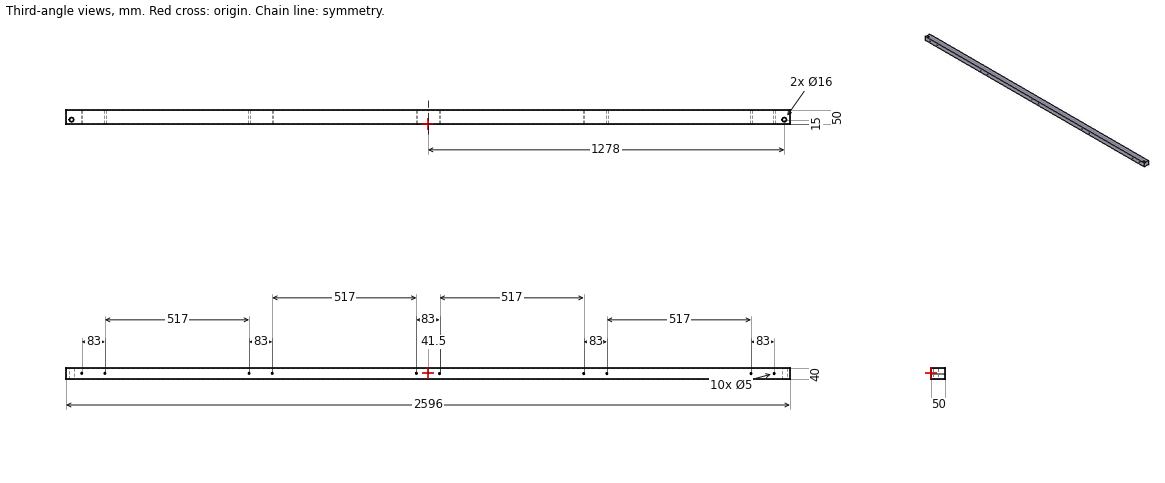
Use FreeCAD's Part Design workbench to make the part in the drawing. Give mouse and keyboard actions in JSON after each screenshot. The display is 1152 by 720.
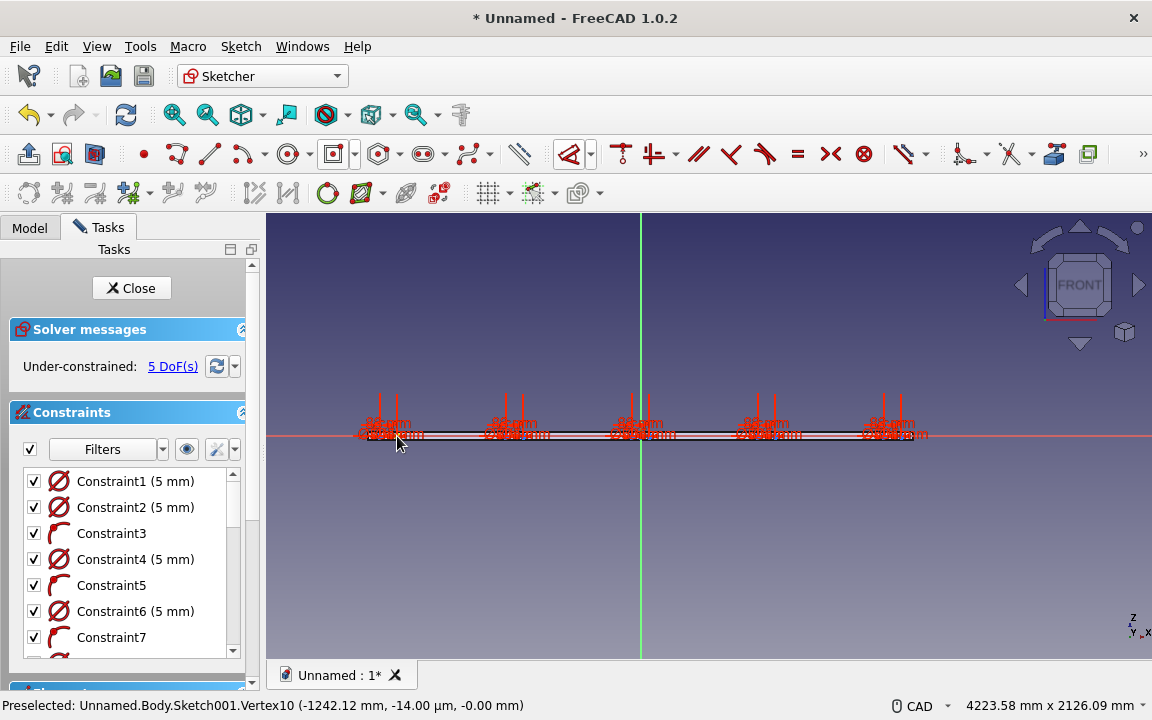
{"action": "scroll", "coordinate": [649, 436], "scroll_direction": "up", "scroll_amount": 8}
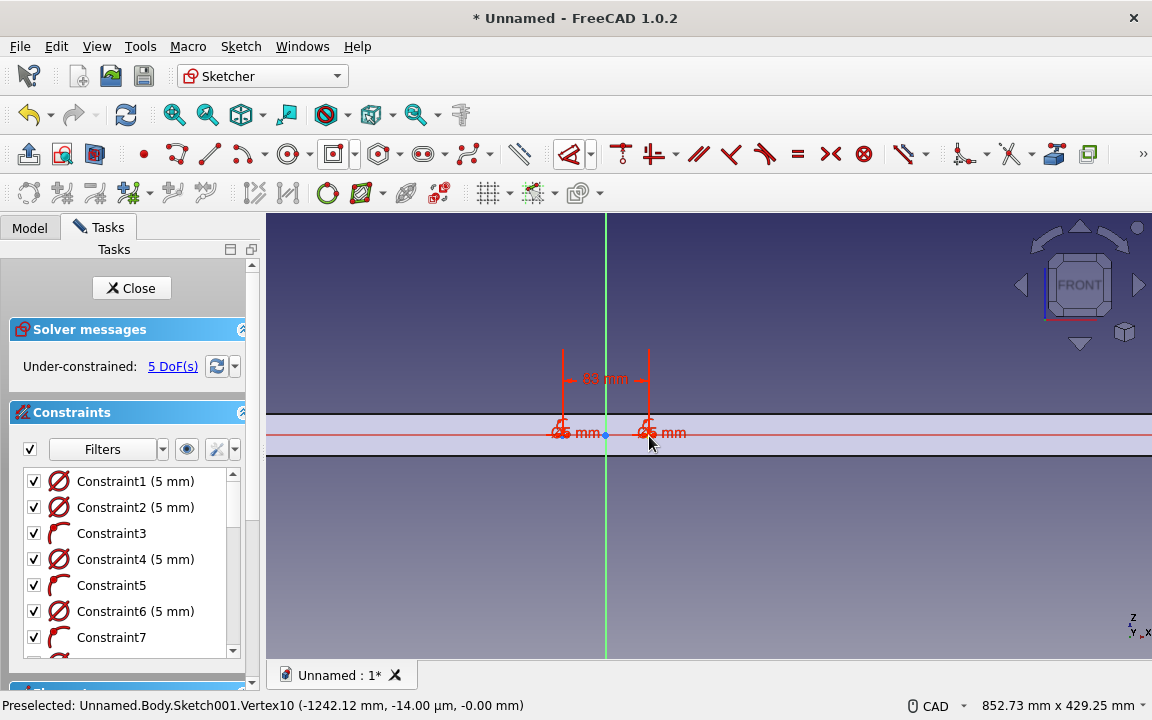
{"action": "left_click", "coordinate": [649, 435]}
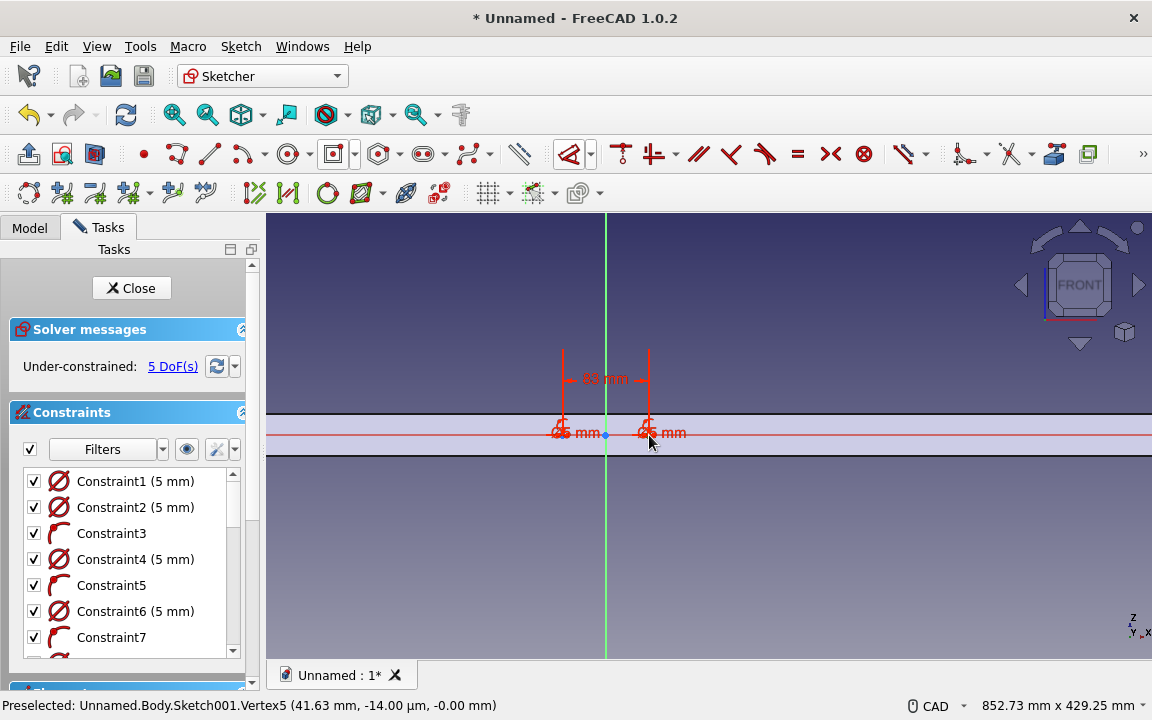
{"action": "left_click", "coordinate": [590, 154]}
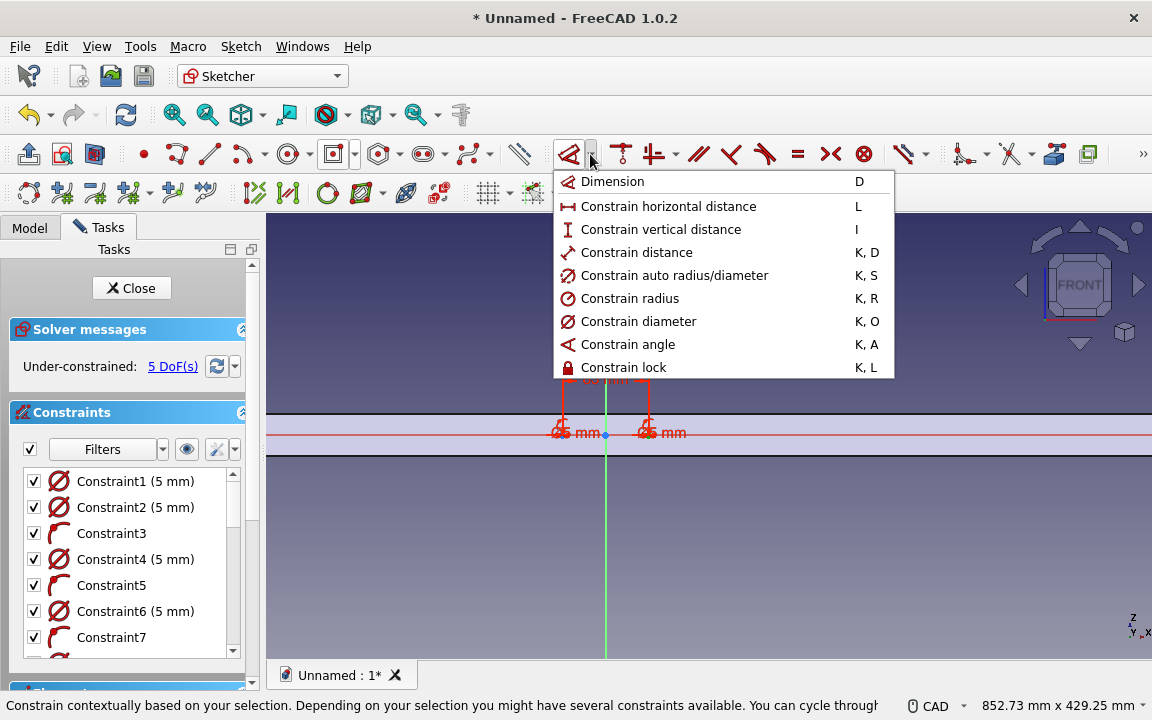
{"action": "left_click", "coordinate": [724, 206]}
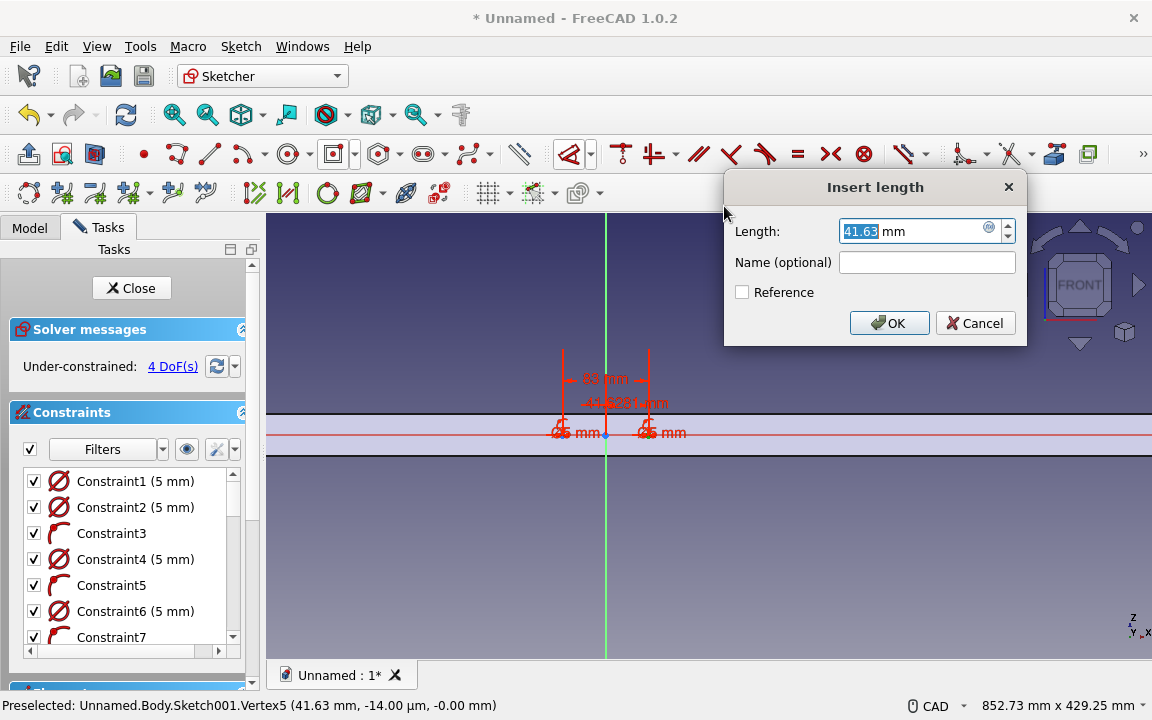
{"action": "type", "text": "41.5"}
{"action": "key", "text": "Return"}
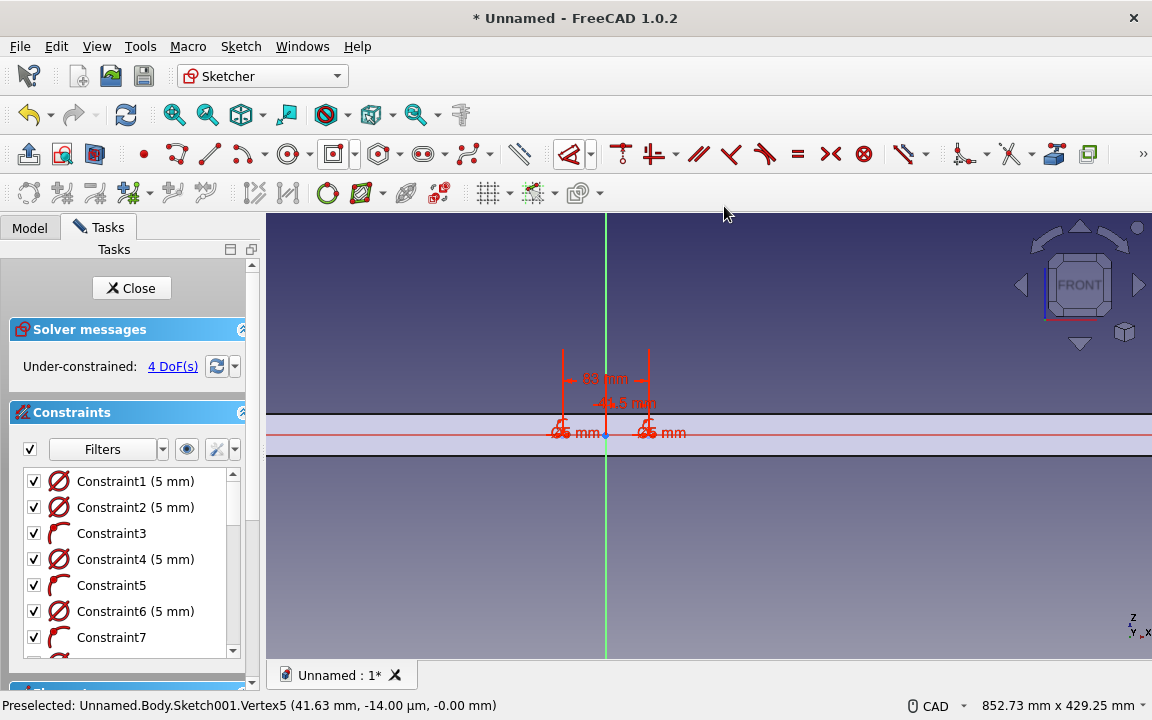
{"action": "scroll", "coordinate": [649, 436], "scroll_direction": "down", "scroll_amount": 8}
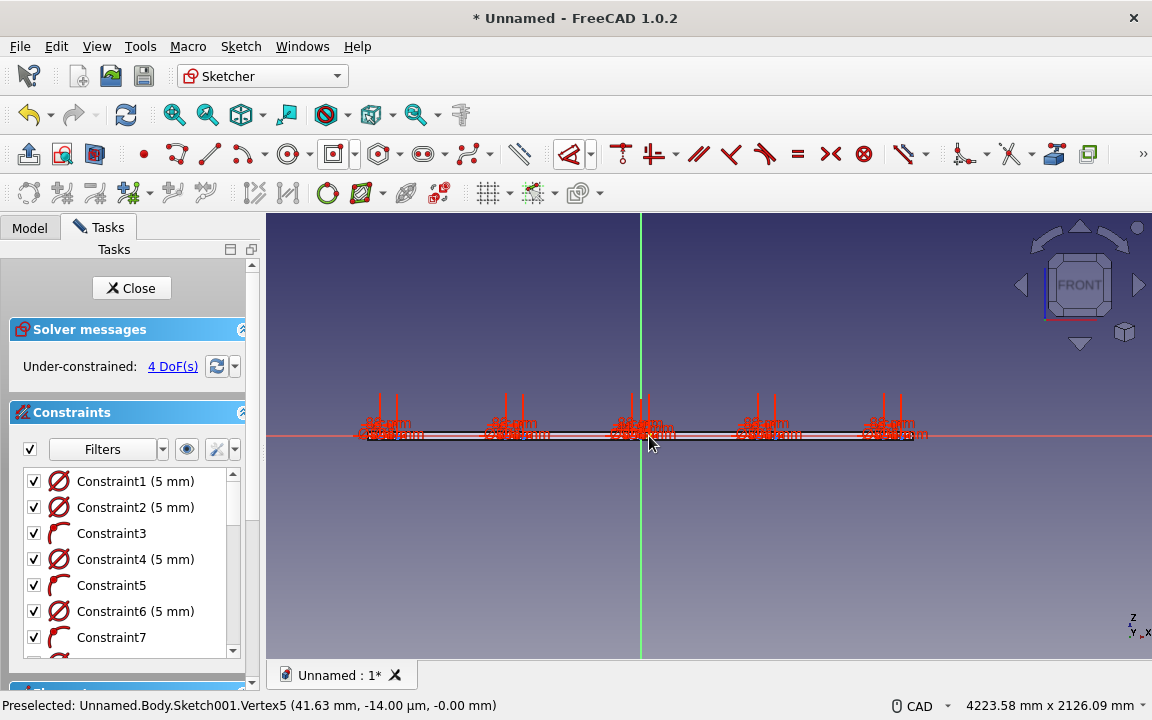
{"action": "left_click", "coordinate": [884, 436]}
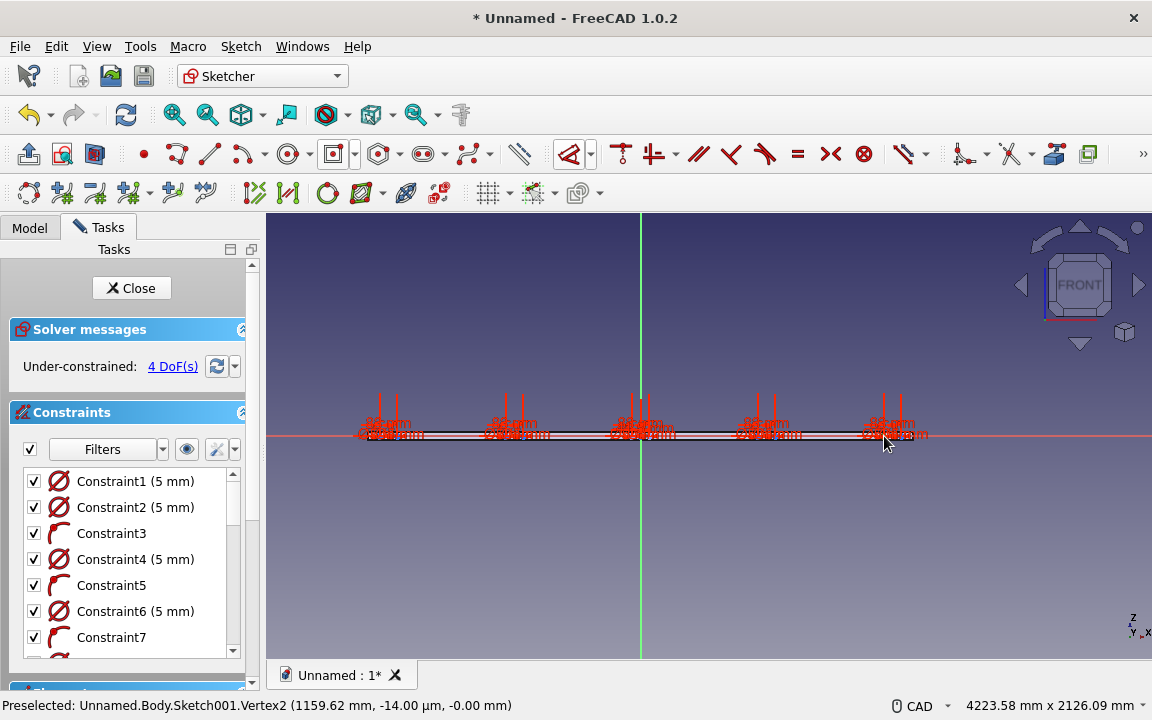
{"action": "left_click", "coordinate": [775, 436]}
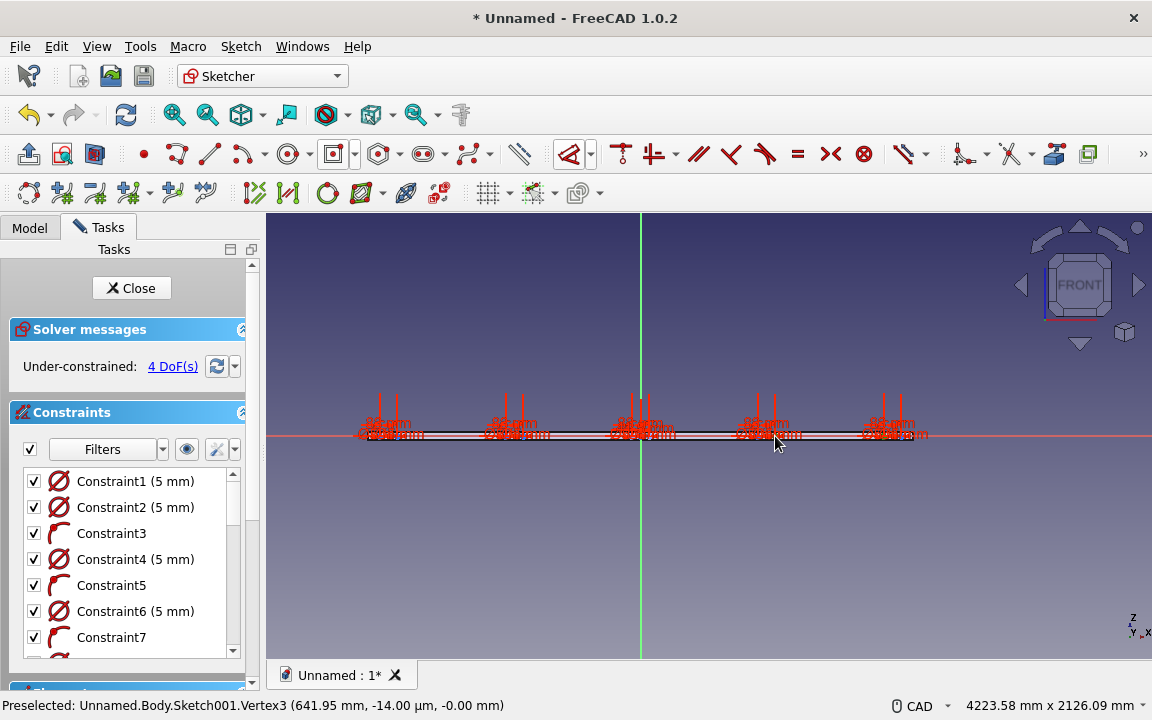
{"action": "left_click", "coordinate": [590, 154]}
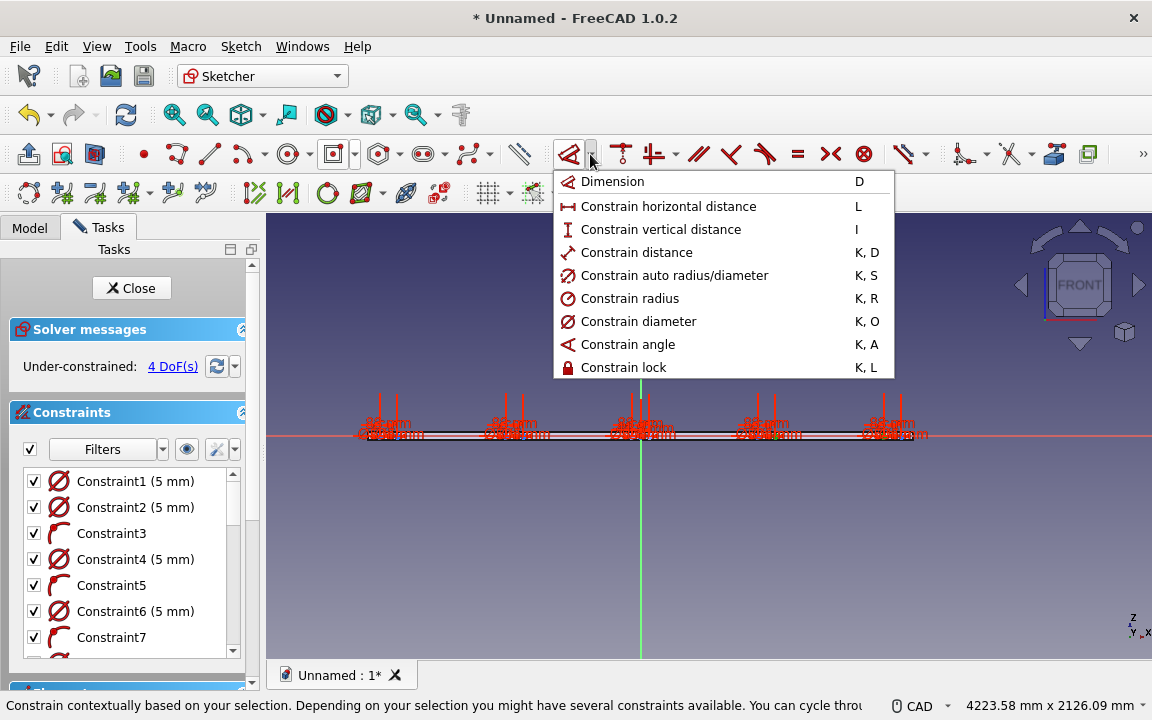
{"action": "left_click", "coordinate": [724, 206]}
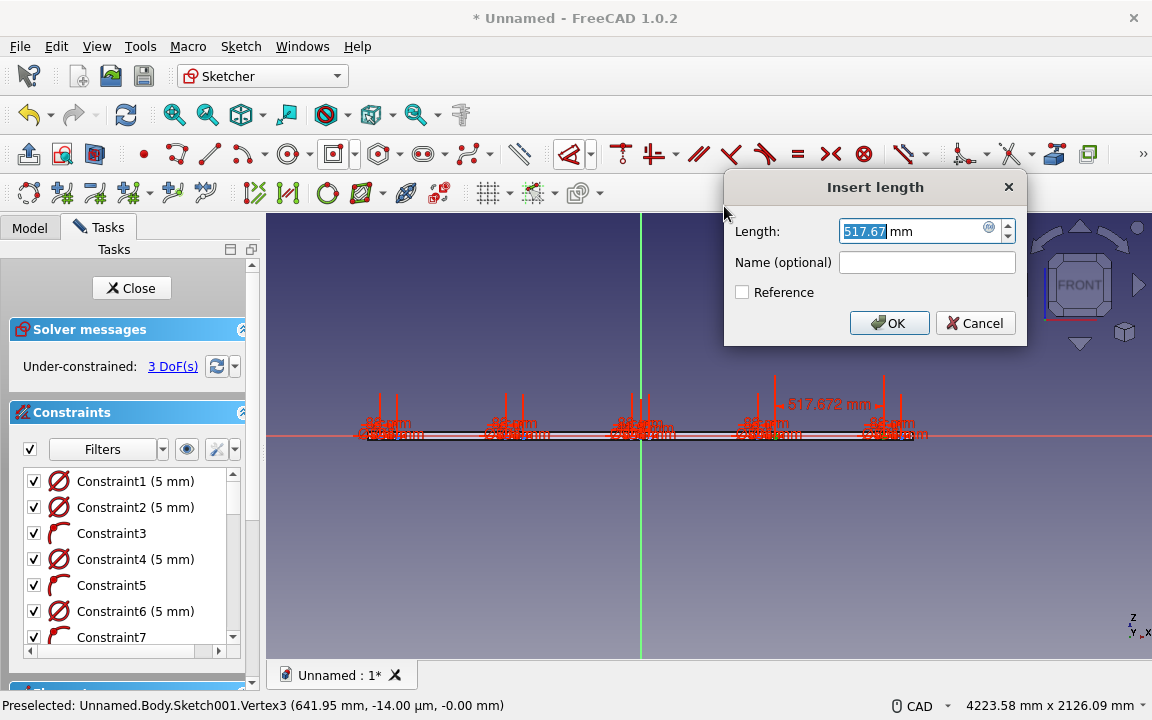
{"action": "type", "text": "517"}
{"action": "key", "text": "Return"}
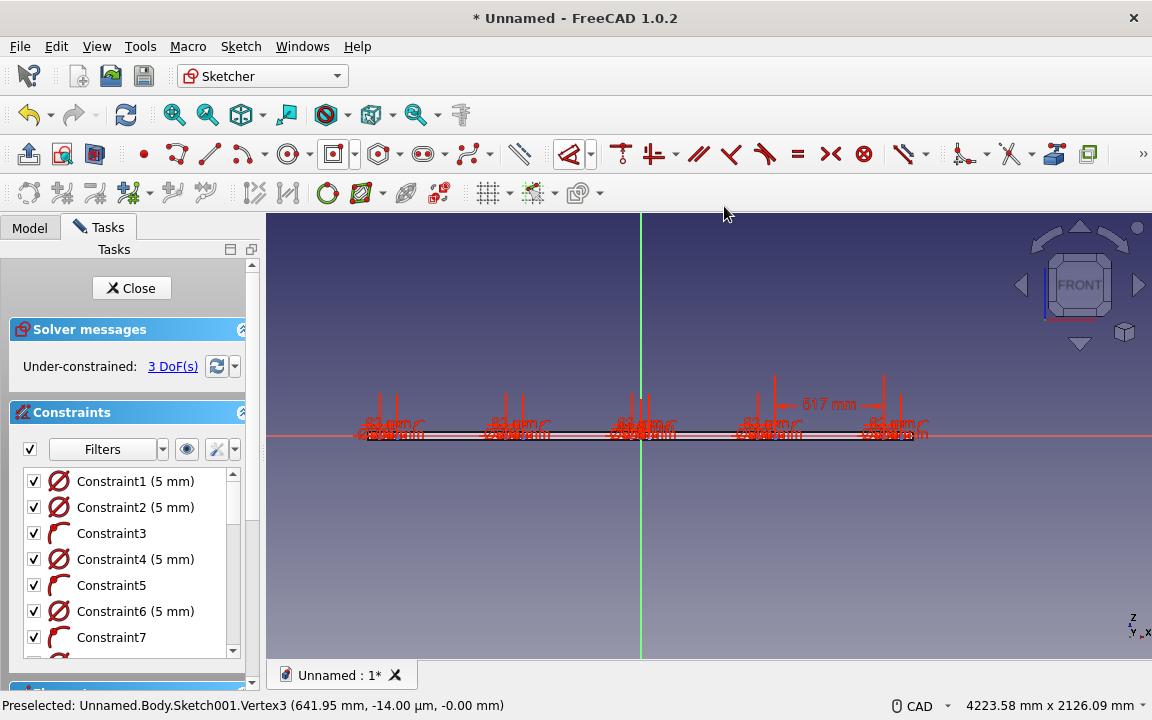
{"action": "left_click", "coordinate": [758, 436]}